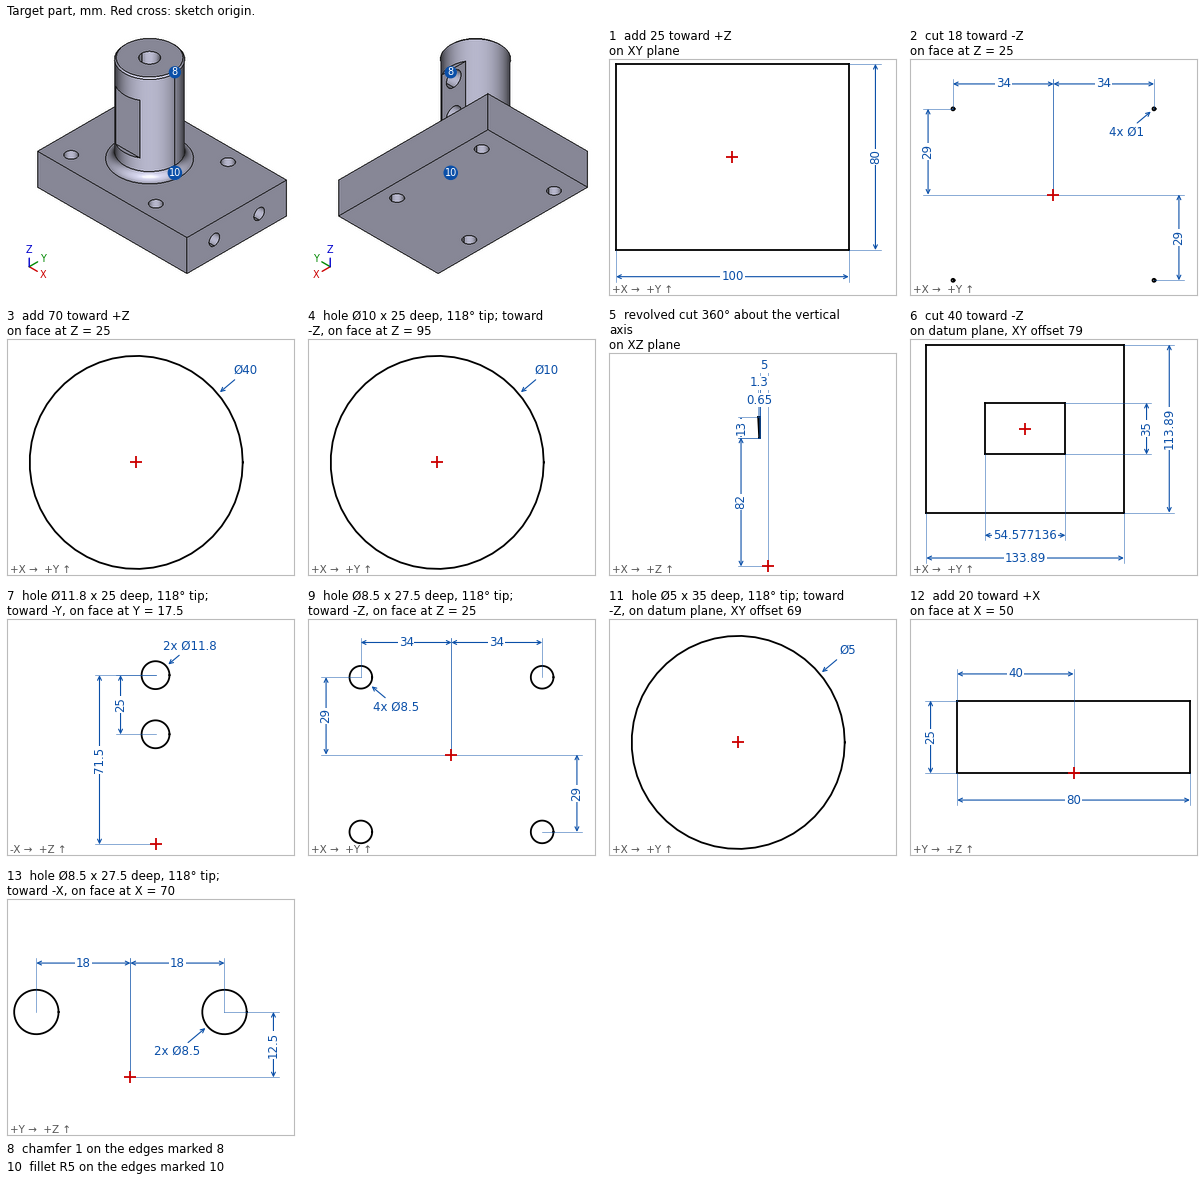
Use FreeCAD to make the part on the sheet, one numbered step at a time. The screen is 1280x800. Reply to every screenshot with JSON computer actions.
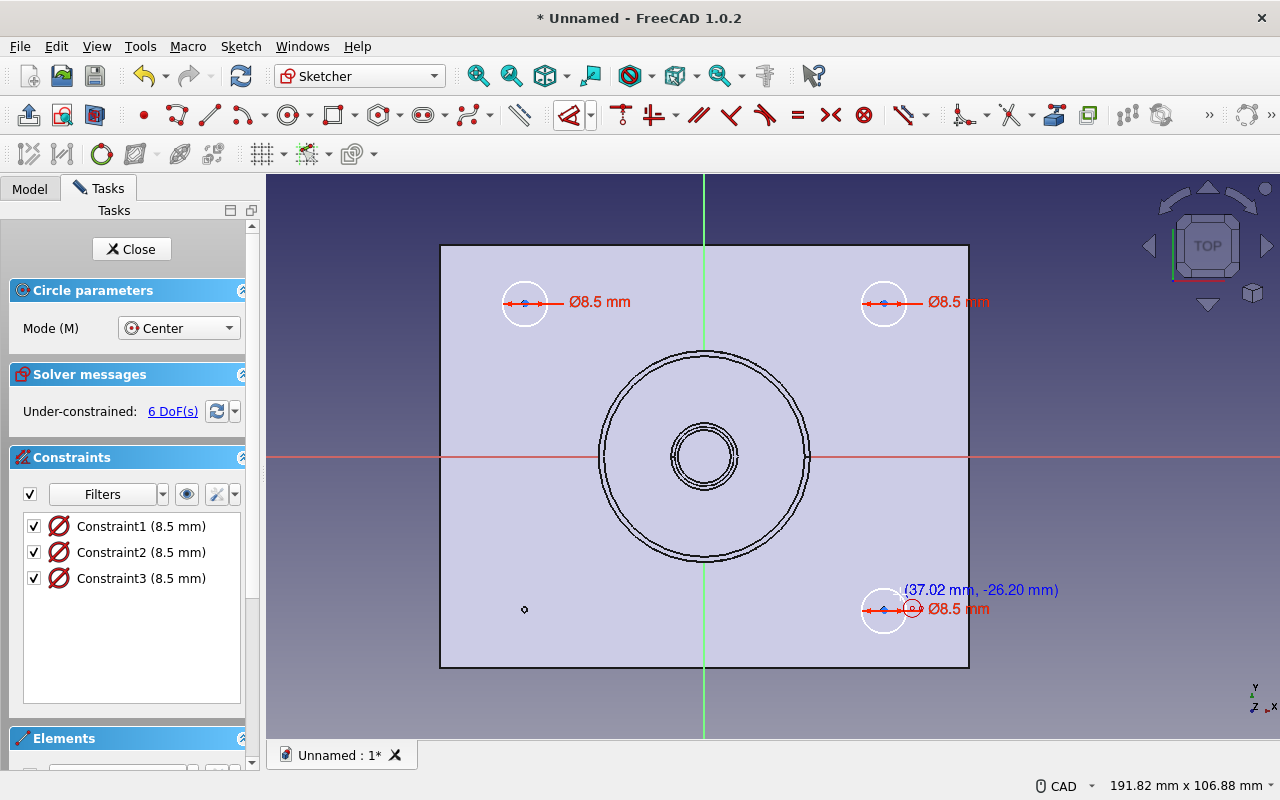
{"action": "left_click", "coordinate": [525, 610]}
{"action": "mouse_move", "coordinate": [540, 594]}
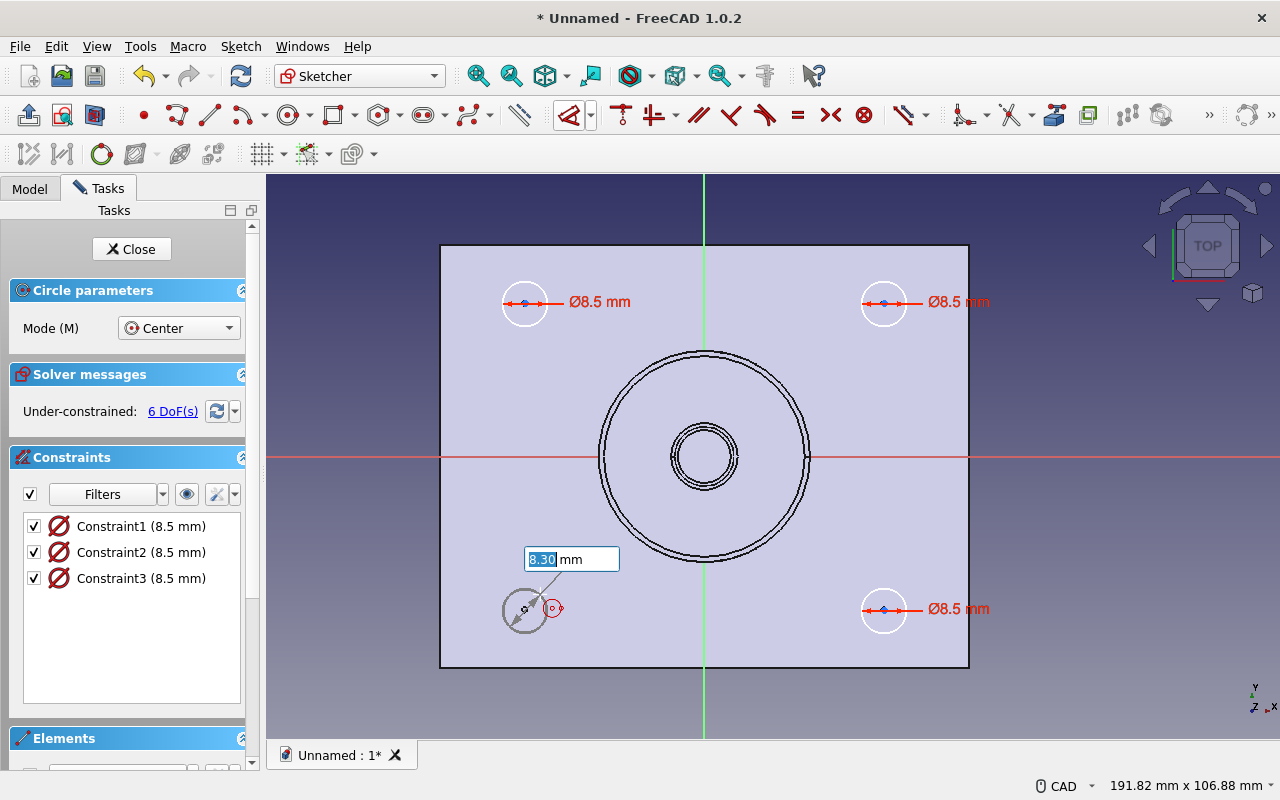
{"action": "type", "text": "8.5"}
{"action": "key", "text": "Return"}
{"action": "key", "text": "Escape"}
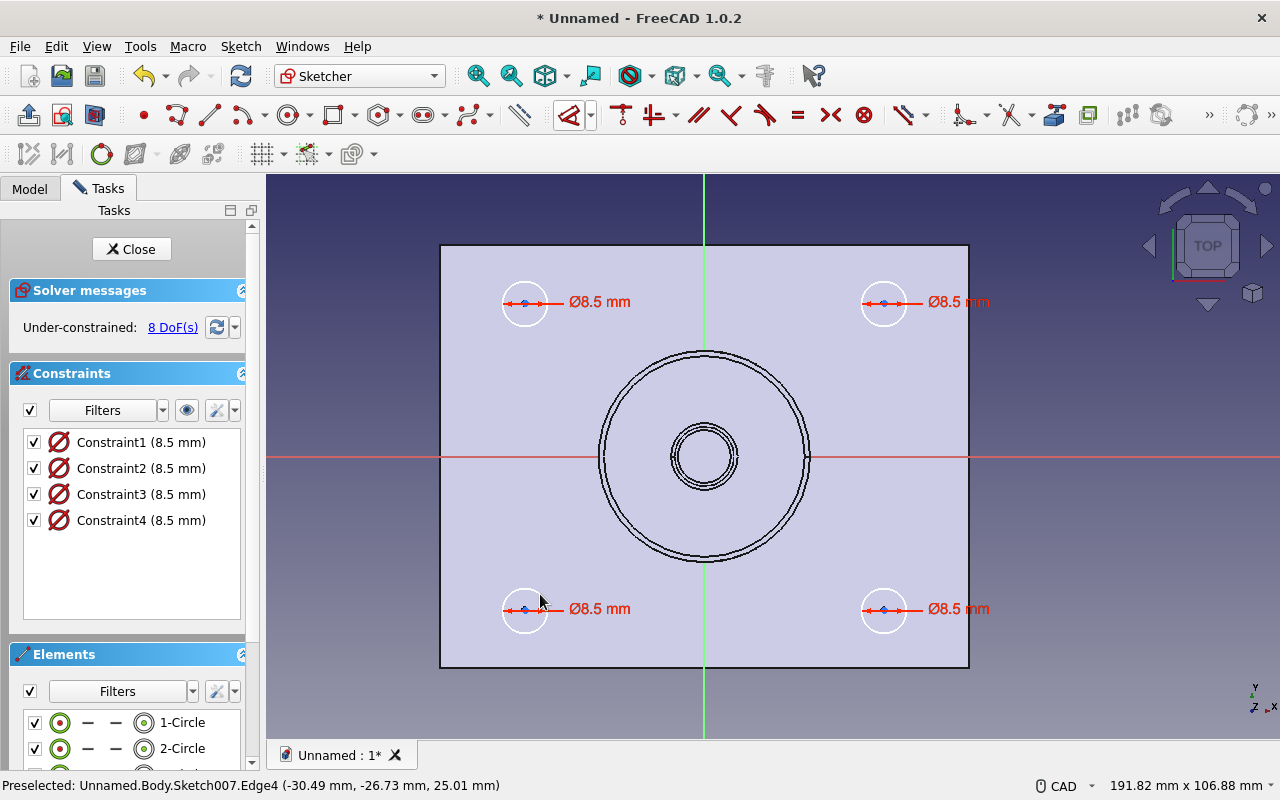
{"action": "left_click", "coordinate": [525, 304]}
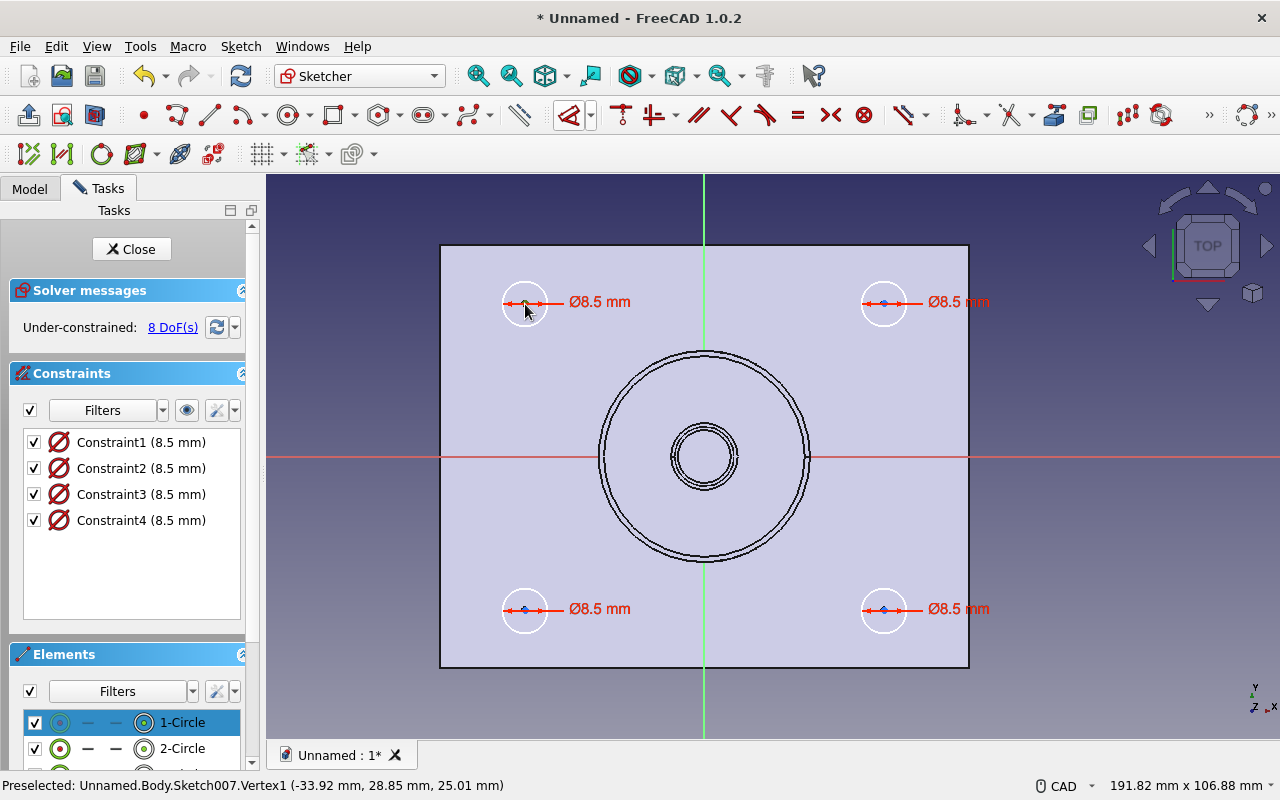
{"action": "left_click", "coordinate": [884, 304]}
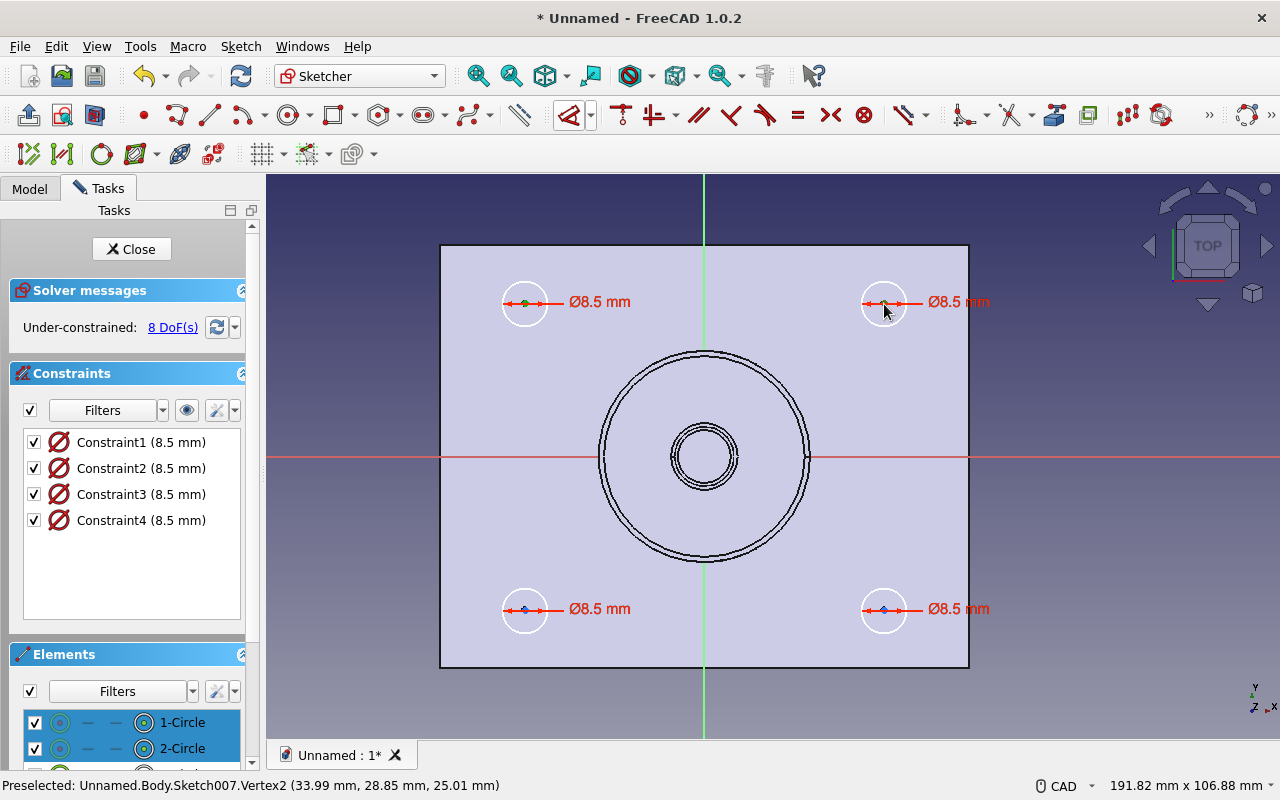
{"action": "key", "text": "h"}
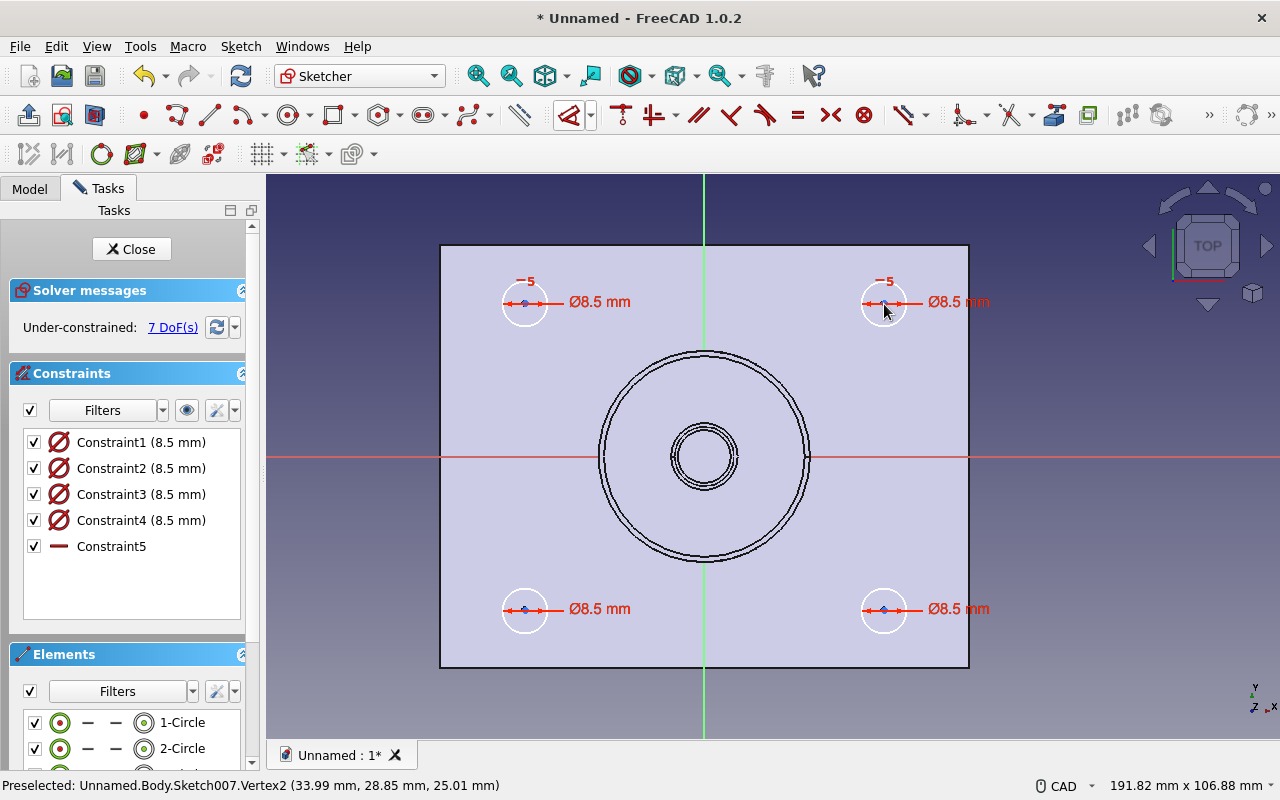
{"action": "left_click", "coordinate": [884, 304]}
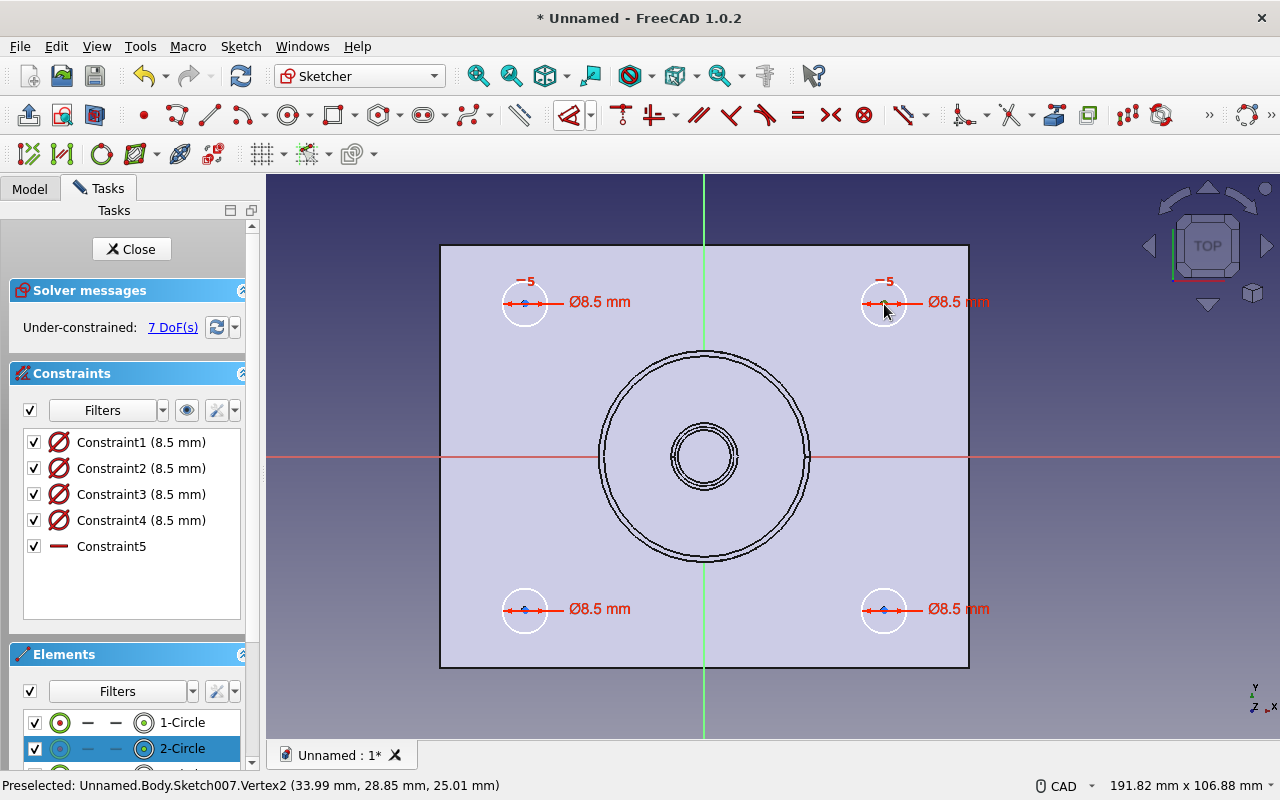
{"action": "left_click", "coordinate": [884, 611]}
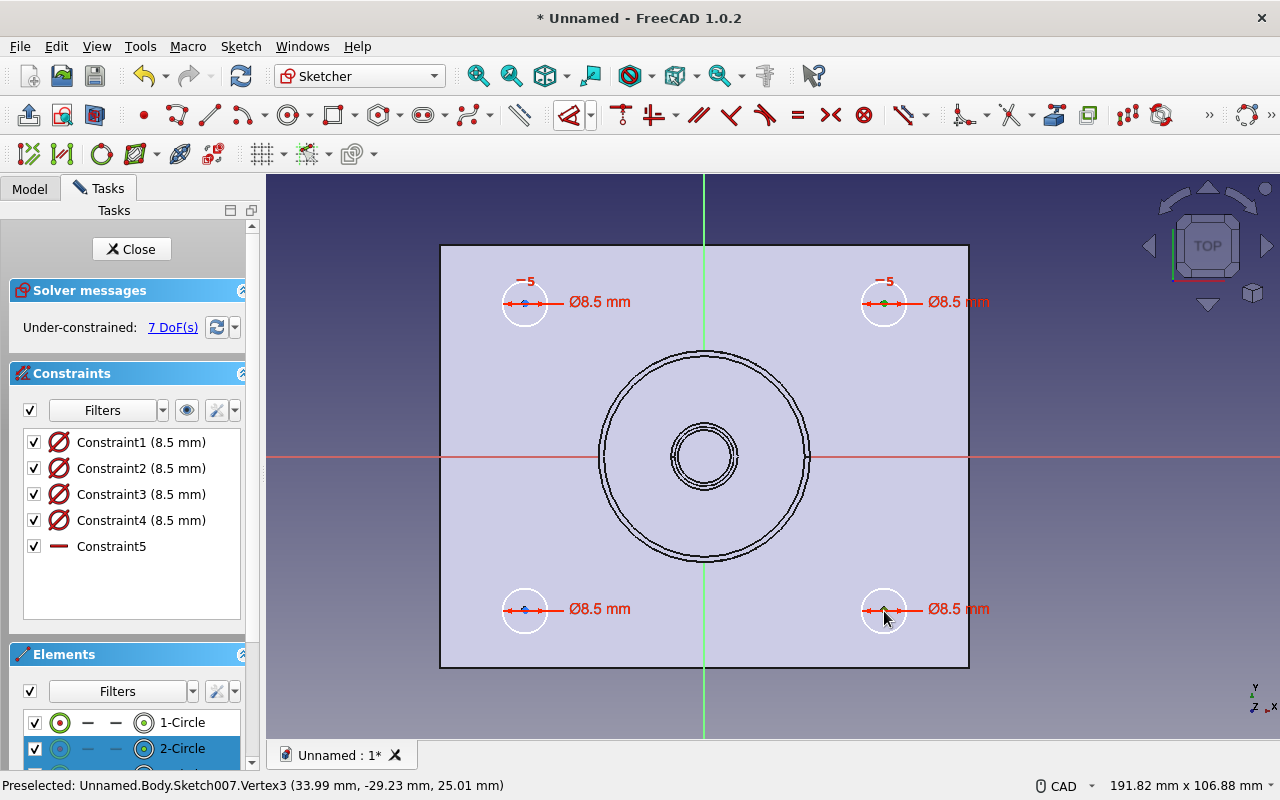
{"action": "key", "text": "v"}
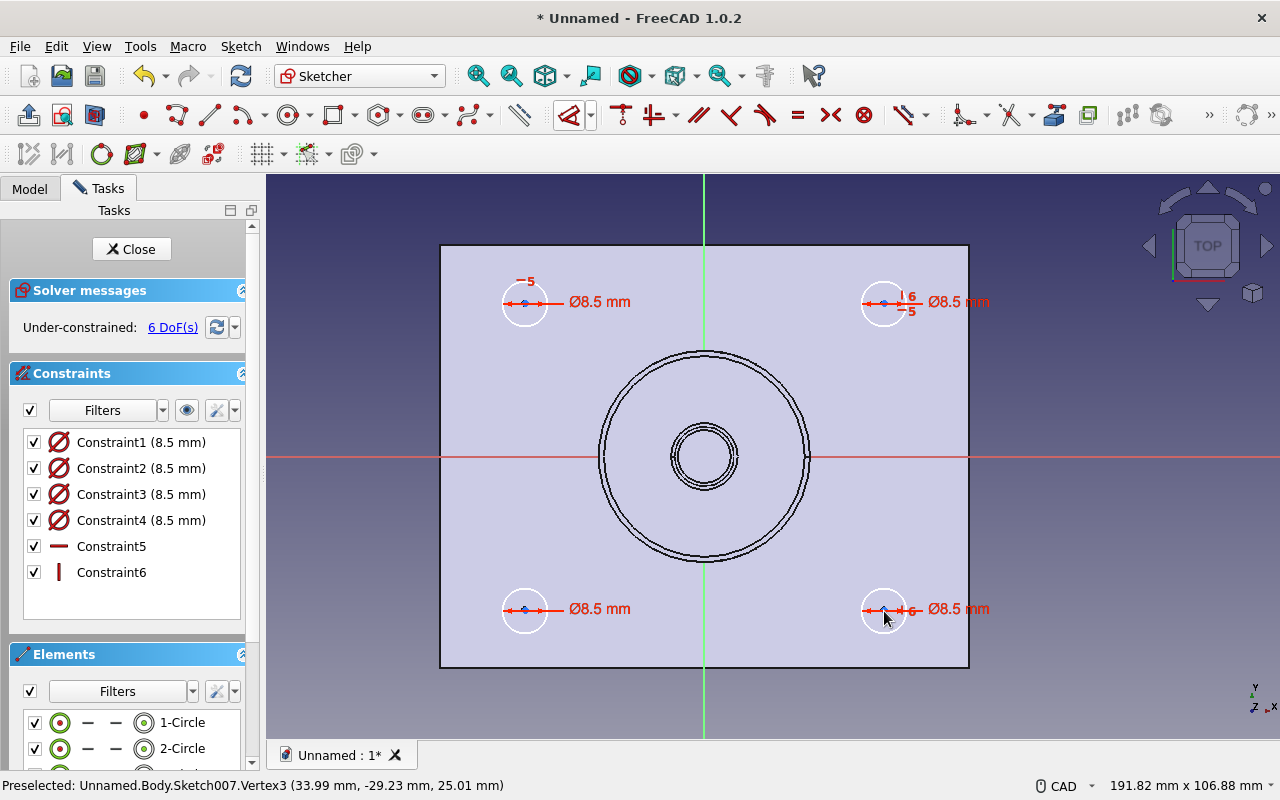
{"action": "left_click", "coordinate": [525, 304]}